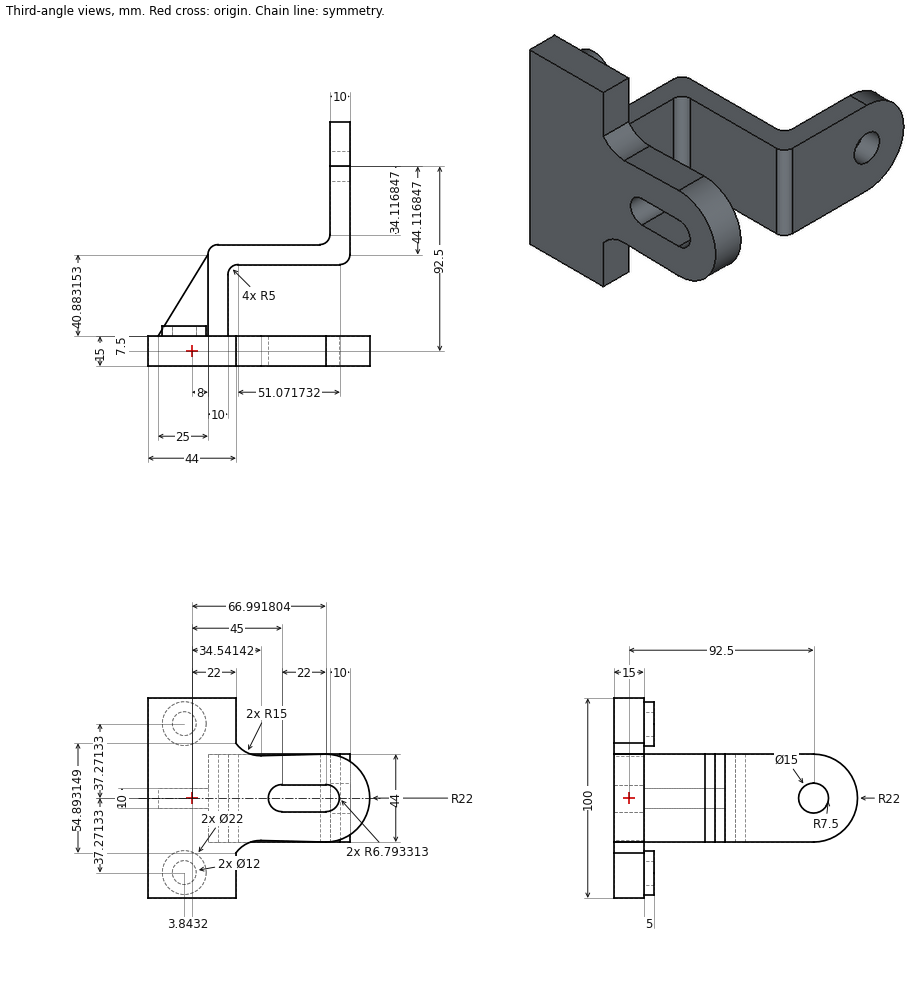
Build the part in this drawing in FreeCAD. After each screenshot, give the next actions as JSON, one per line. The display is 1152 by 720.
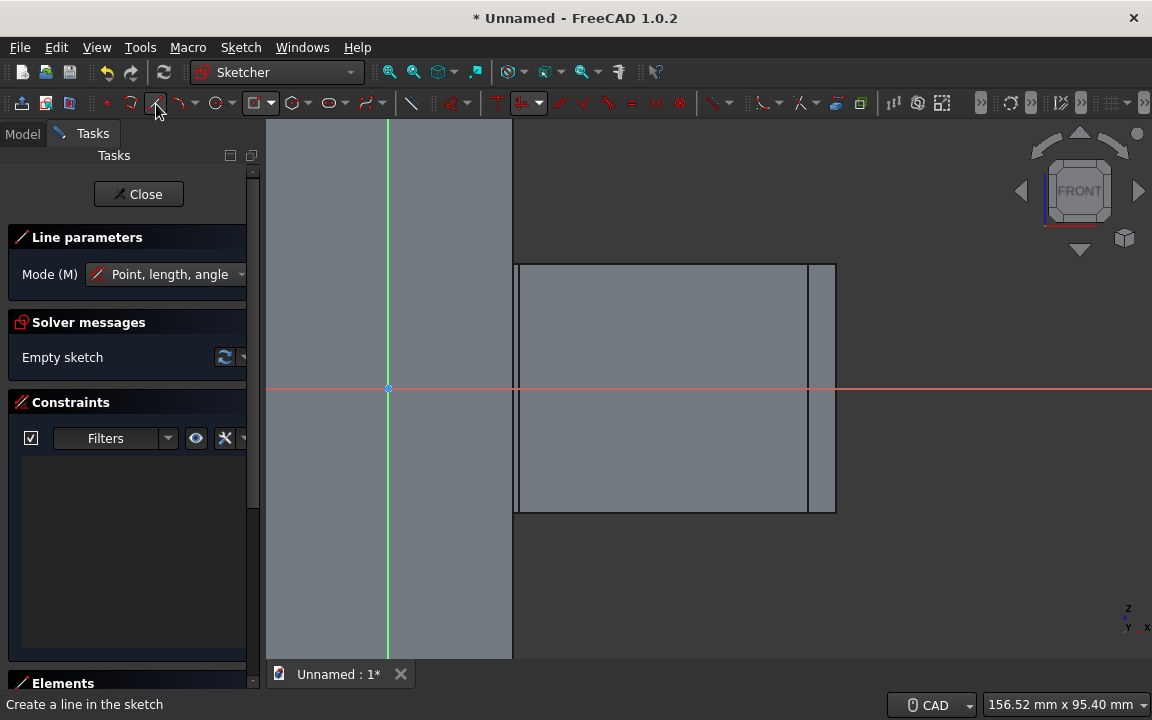
{"action": "left_click", "coordinate": [768, 264]}
{"action": "left_click", "coordinate": [584, 274]}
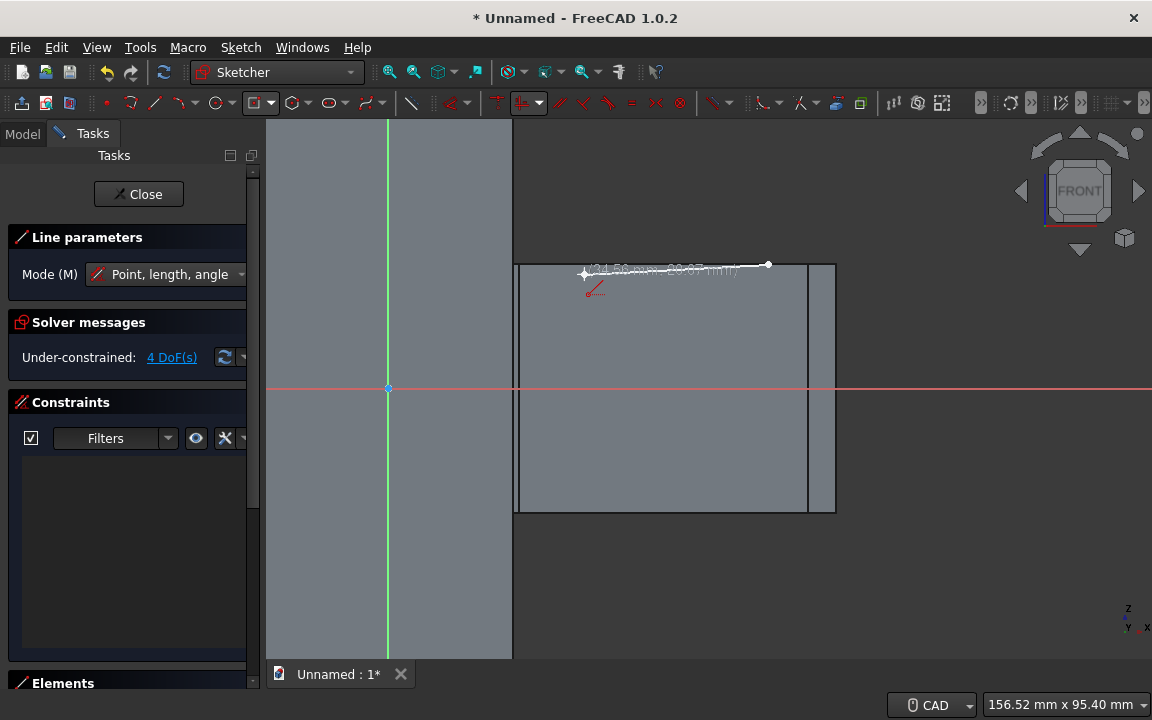
{"action": "left_click", "coordinate": [513, 233]}
{"action": "left_click", "coordinate": [513, 544]}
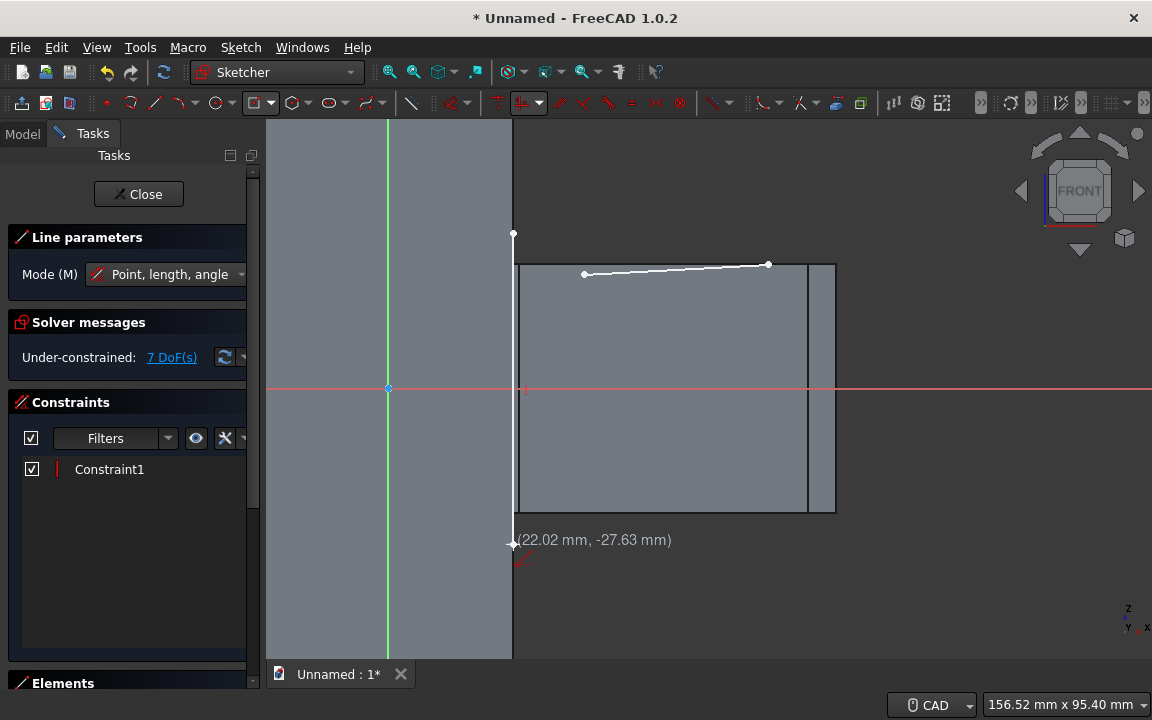
{"action": "left_click", "coordinate": [584, 509]}
{"action": "left_click", "coordinate": [768, 519]}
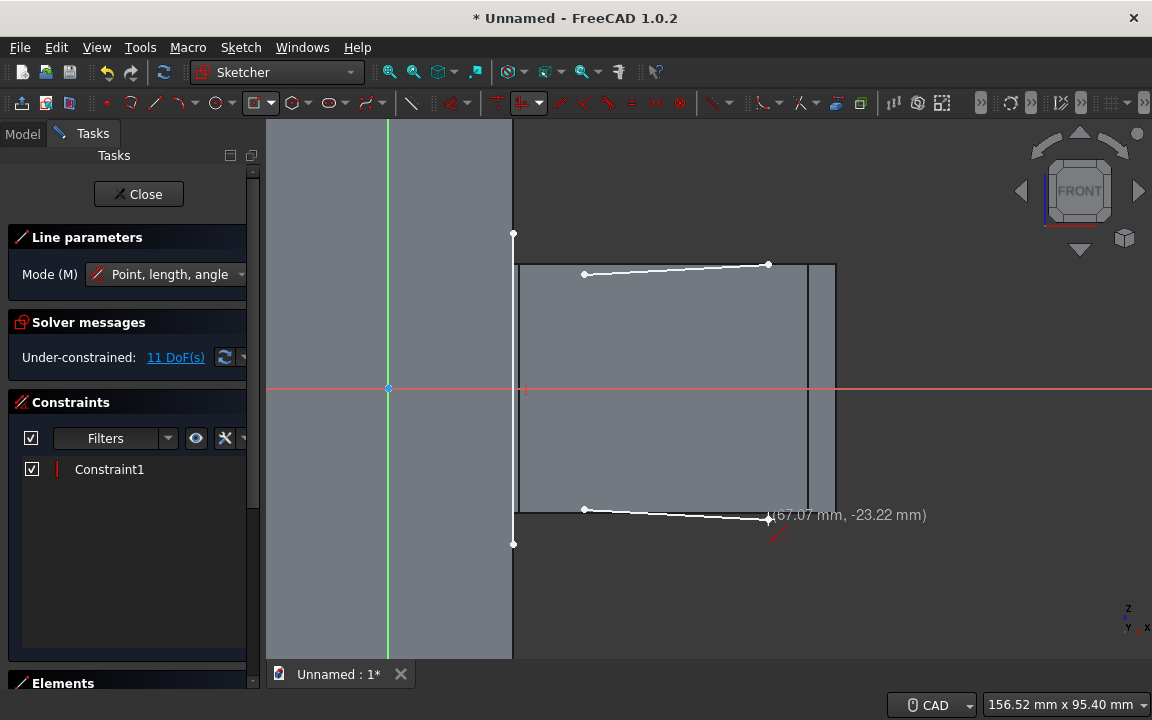
{"action": "left_click", "coordinate": [180, 104]}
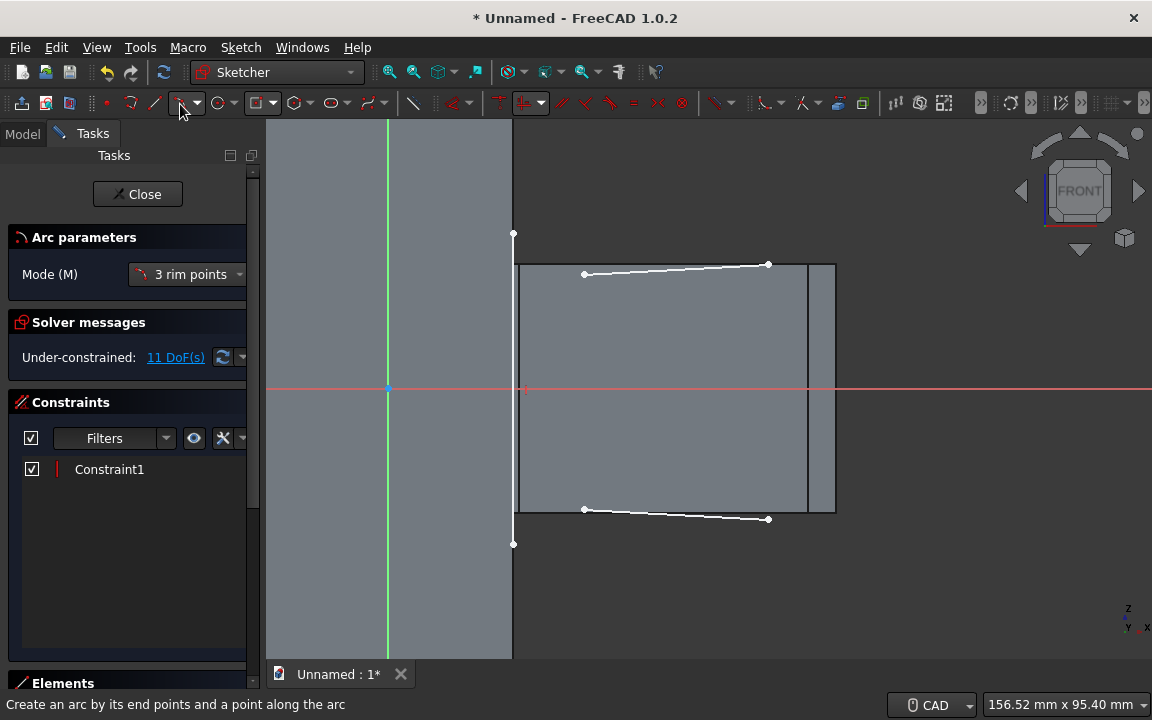
{"action": "left_click", "coordinate": [584, 275]}
{"action": "left_click", "coordinate": [513, 234]}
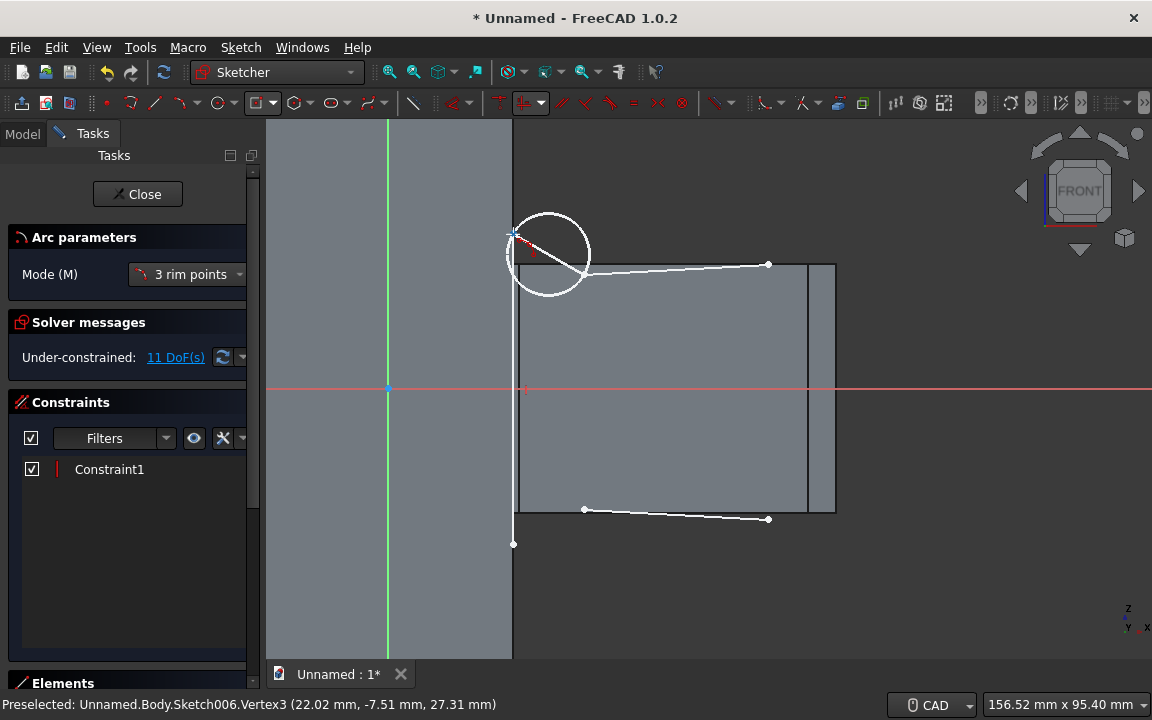
{"action": "scroll", "coordinate": [544, 260], "scroll_direction": "up", "scroll_amount": 3}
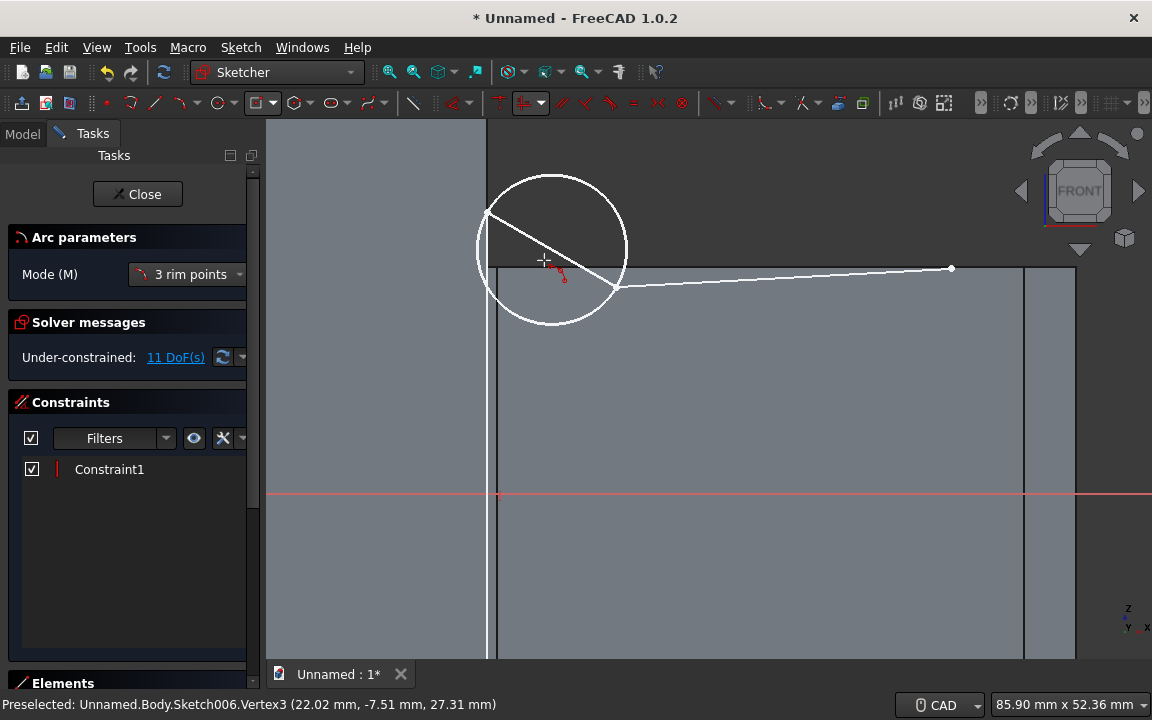
{"action": "left_click", "coordinate": [544, 259]}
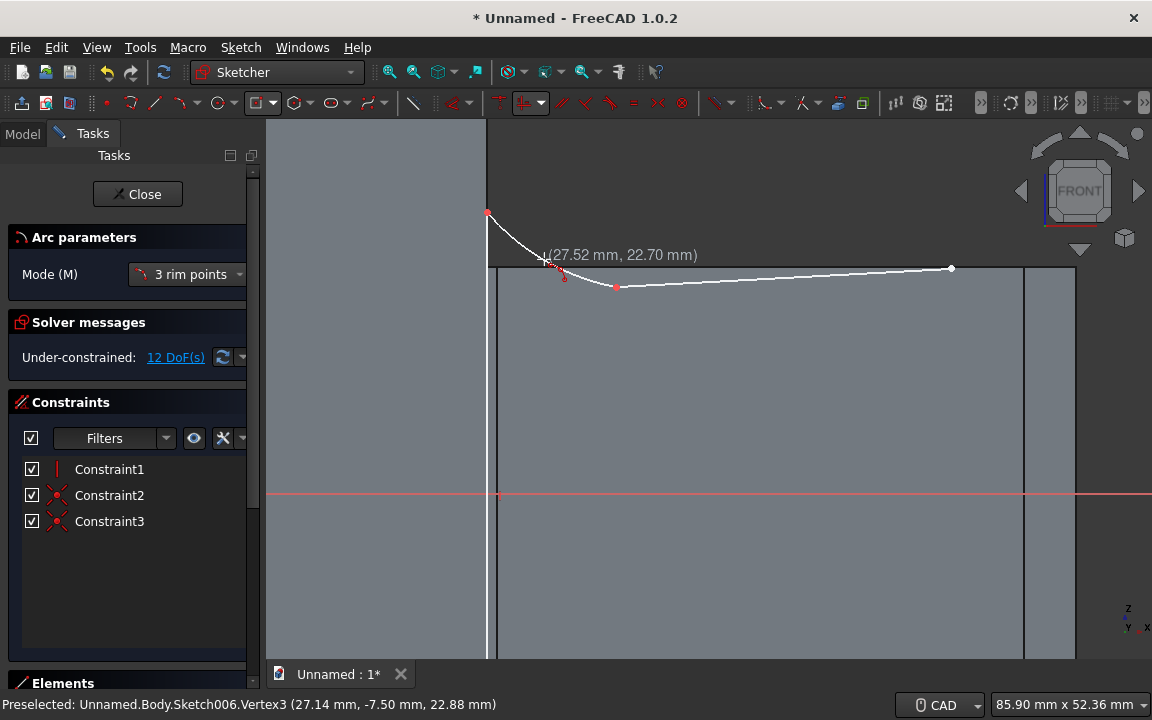
{"action": "scroll", "coordinate": [545, 261], "scroll_direction": "down", "scroll_amount": 3}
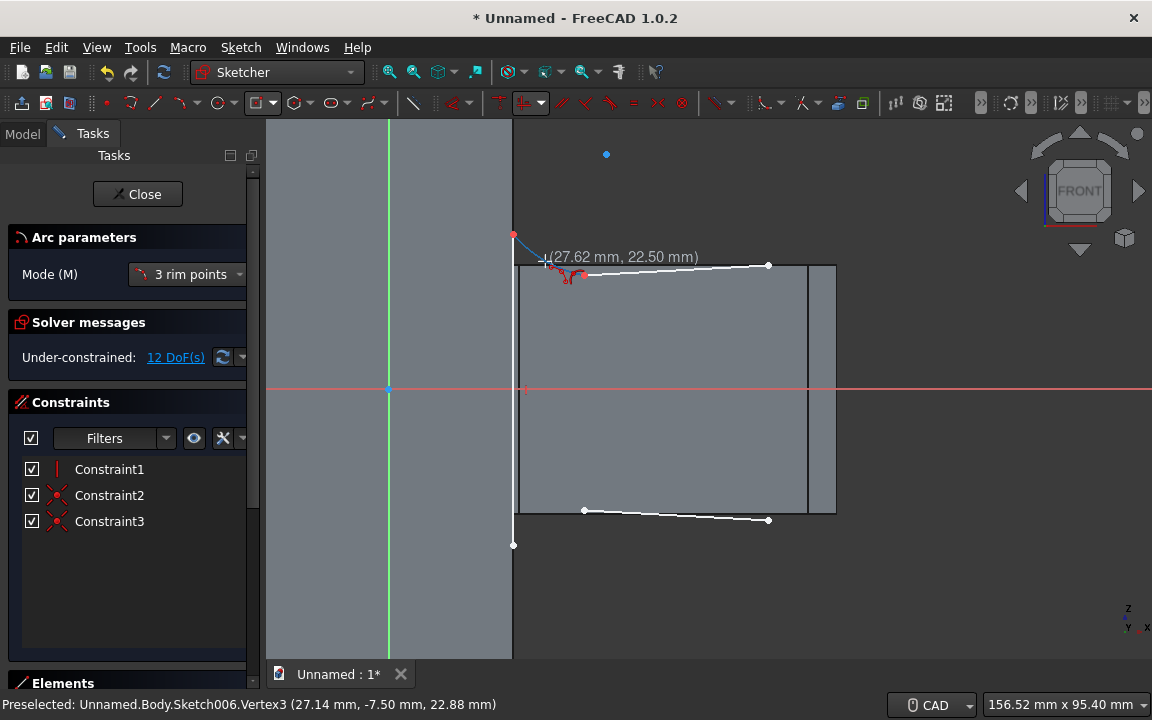
{"action": "left_click", "coordinate": [513, 545]}
{"action": "left_click", "coordinate": [584, 510]}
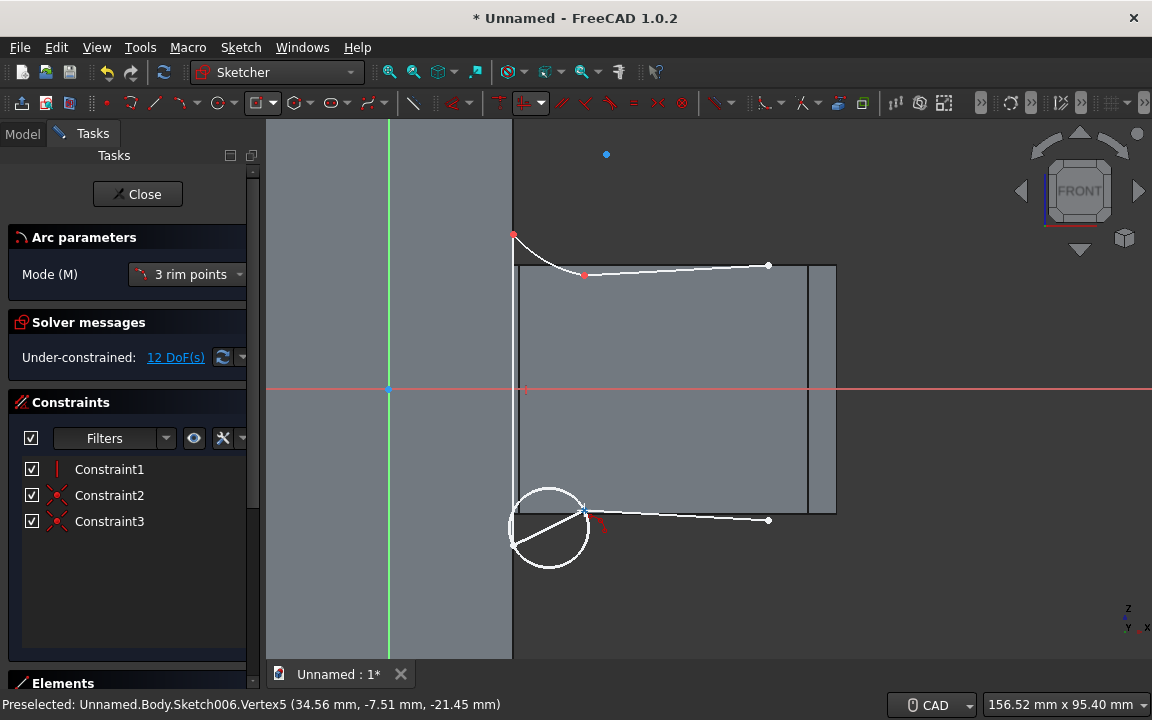
{"action": "scroll", "coordinate": [544, 518], "scroll_direction": "up", "scroll_amount": 3}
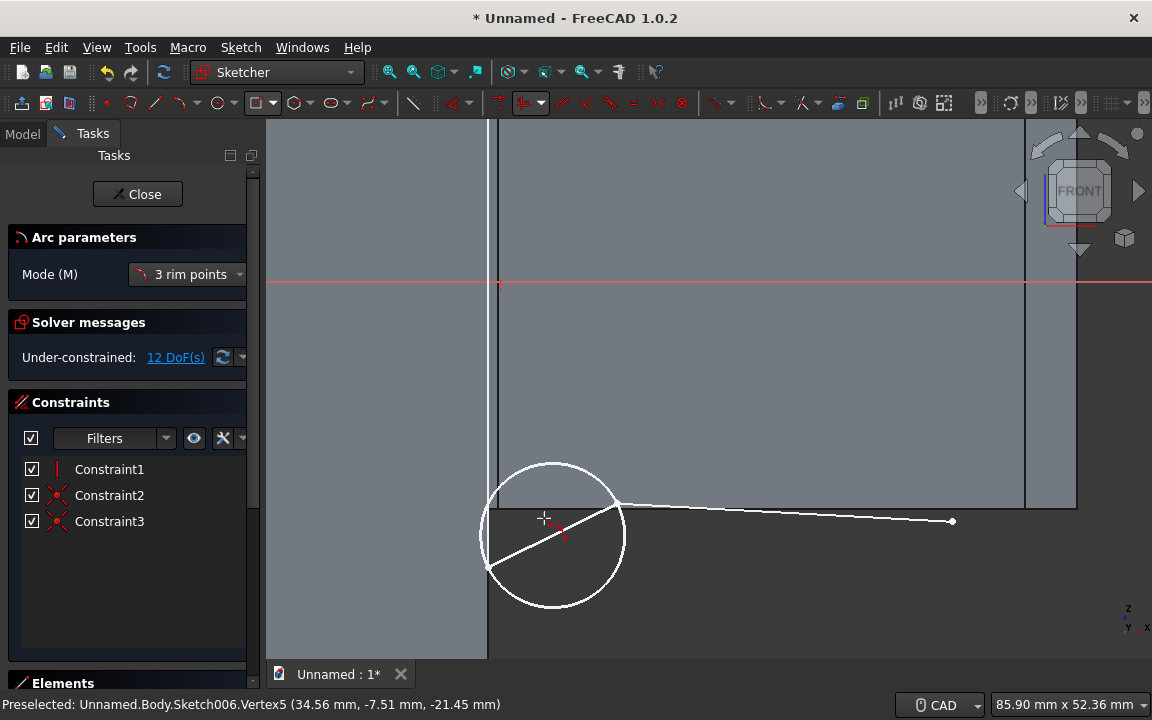
{"action": "left_click", "coordinate": [545, 517]}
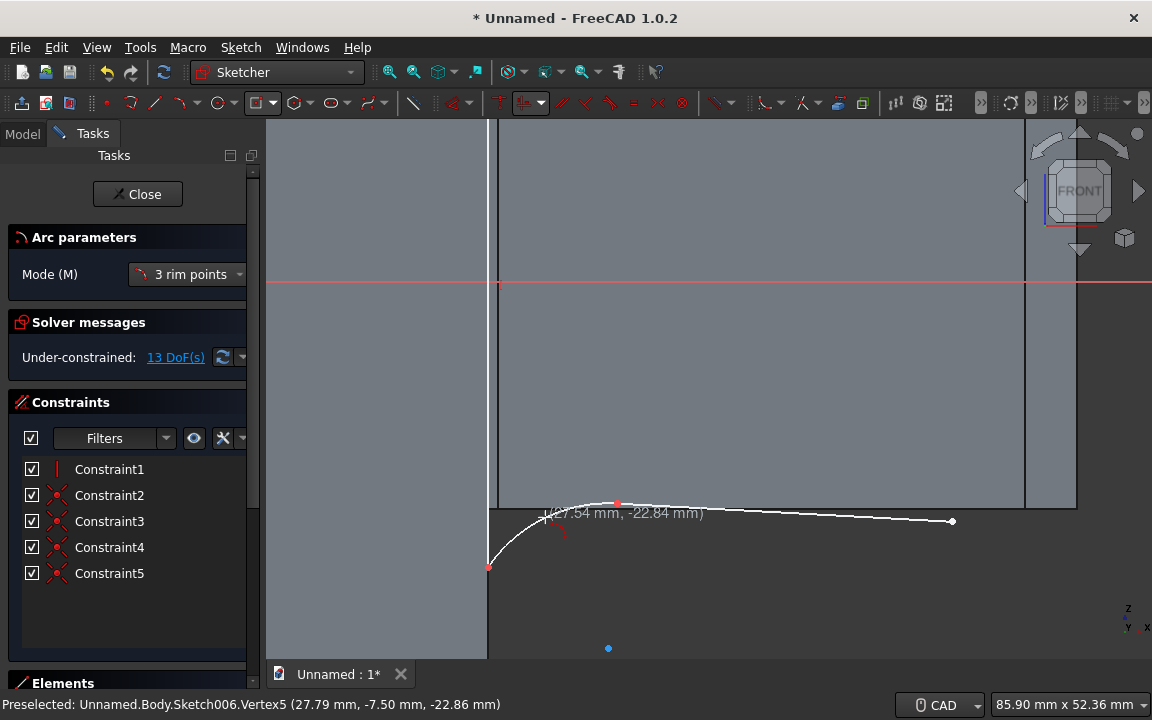
{"action": "left_click", "coordinate": [953, 522]}